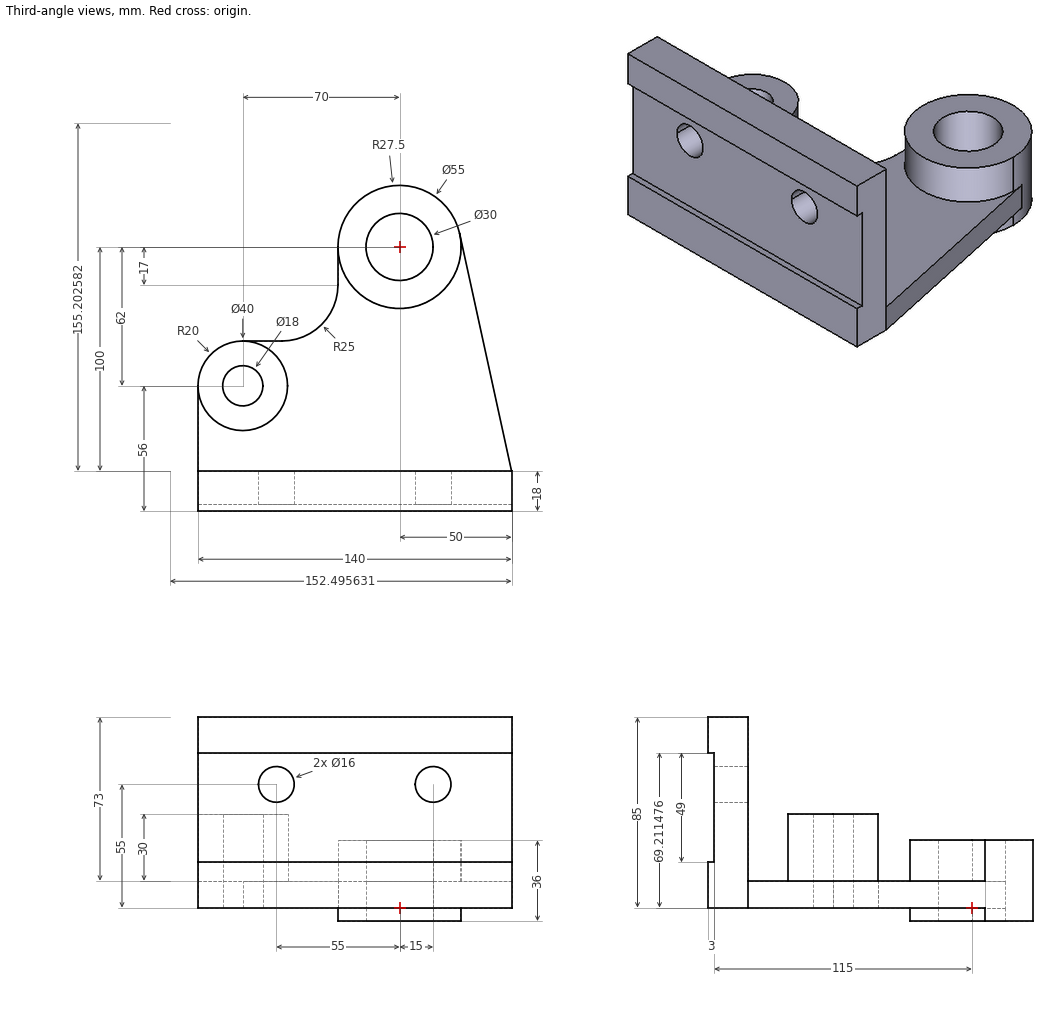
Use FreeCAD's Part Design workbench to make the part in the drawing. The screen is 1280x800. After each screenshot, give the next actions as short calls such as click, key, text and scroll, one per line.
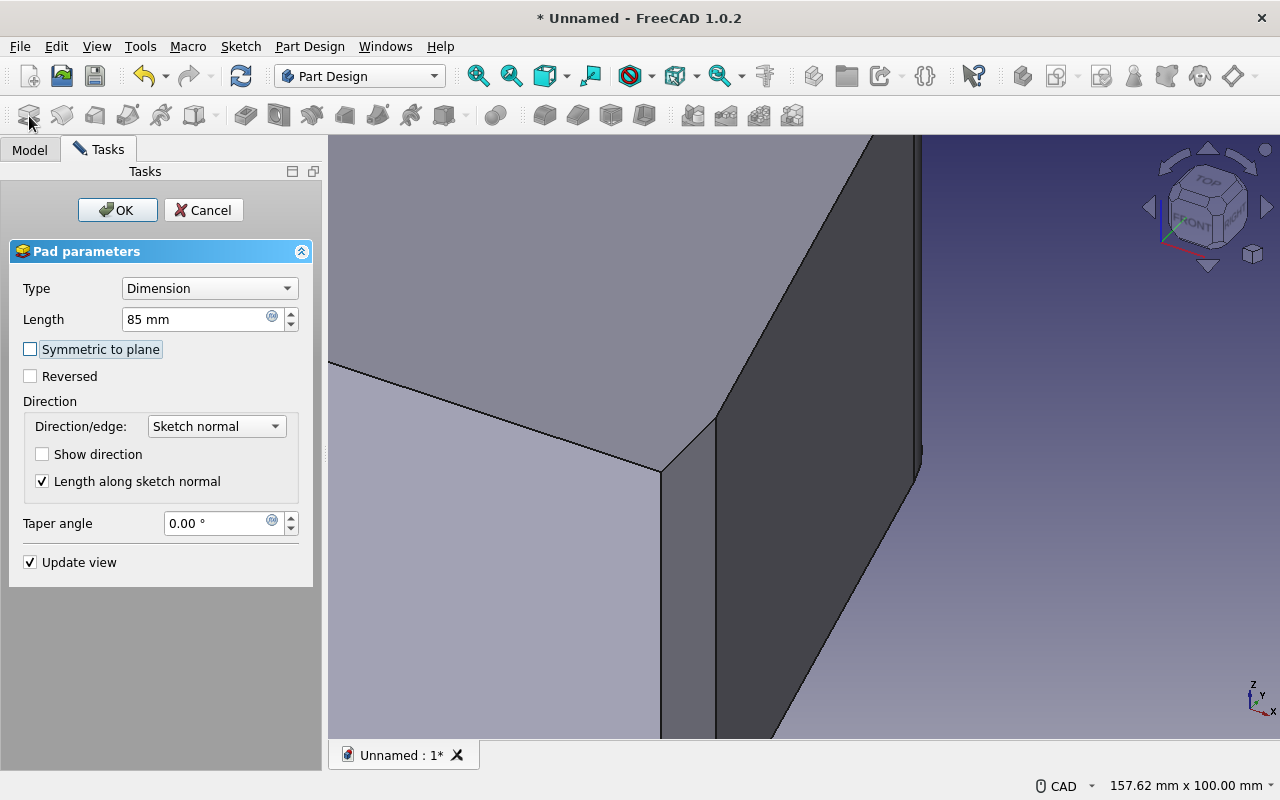
click(118, 210)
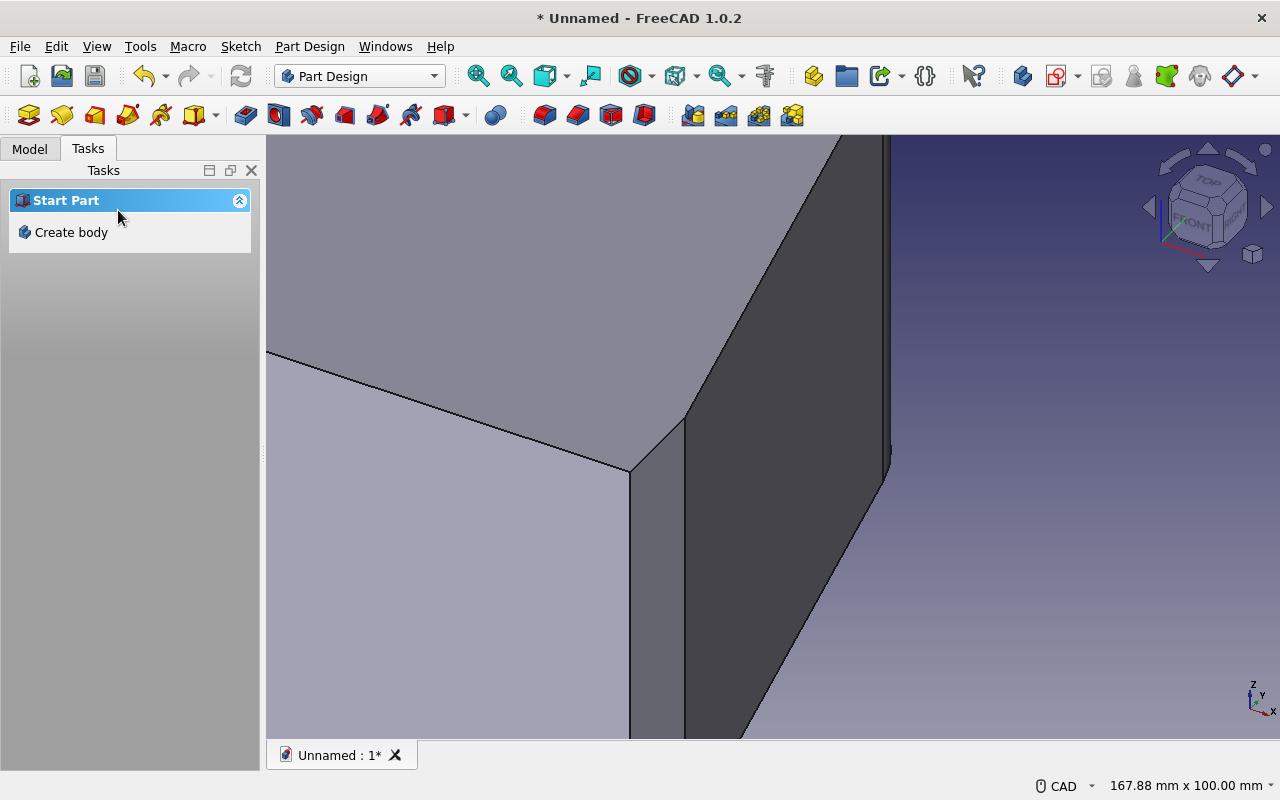
click(479, 76)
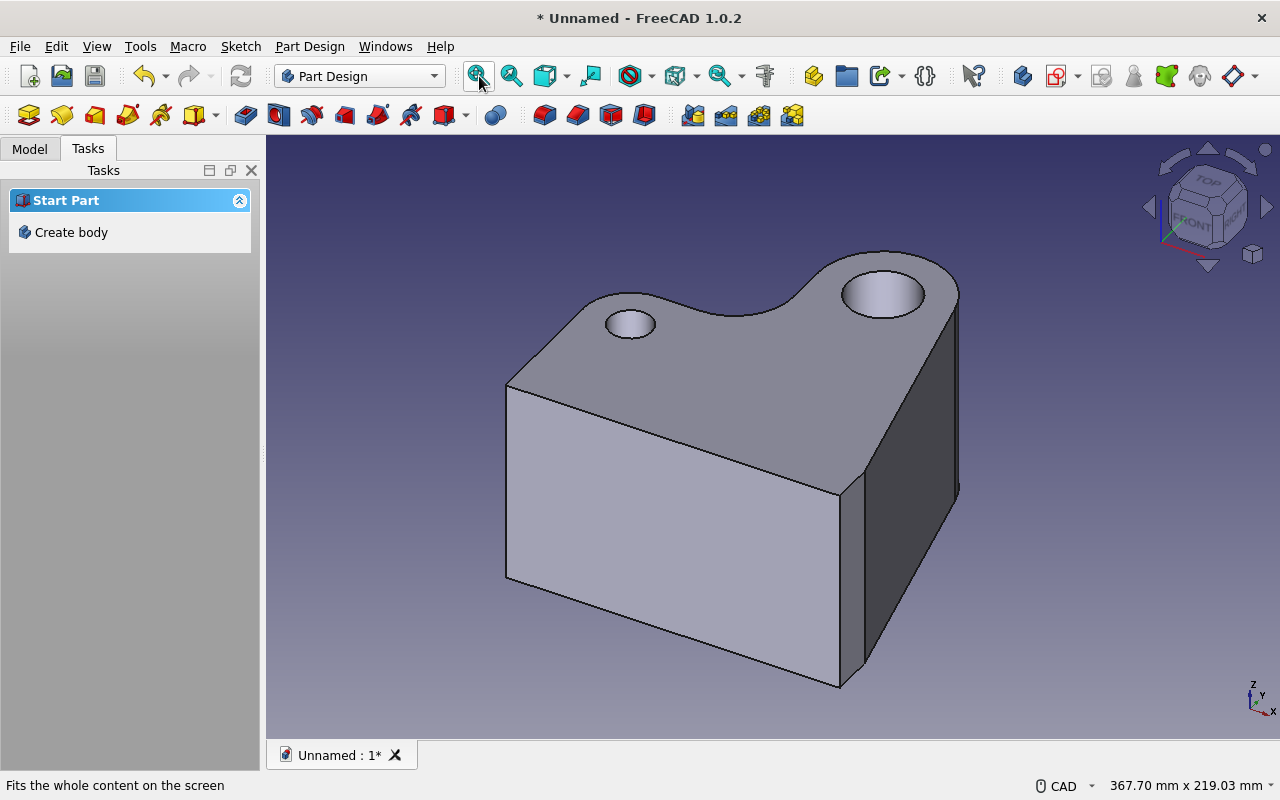
click(792, 384)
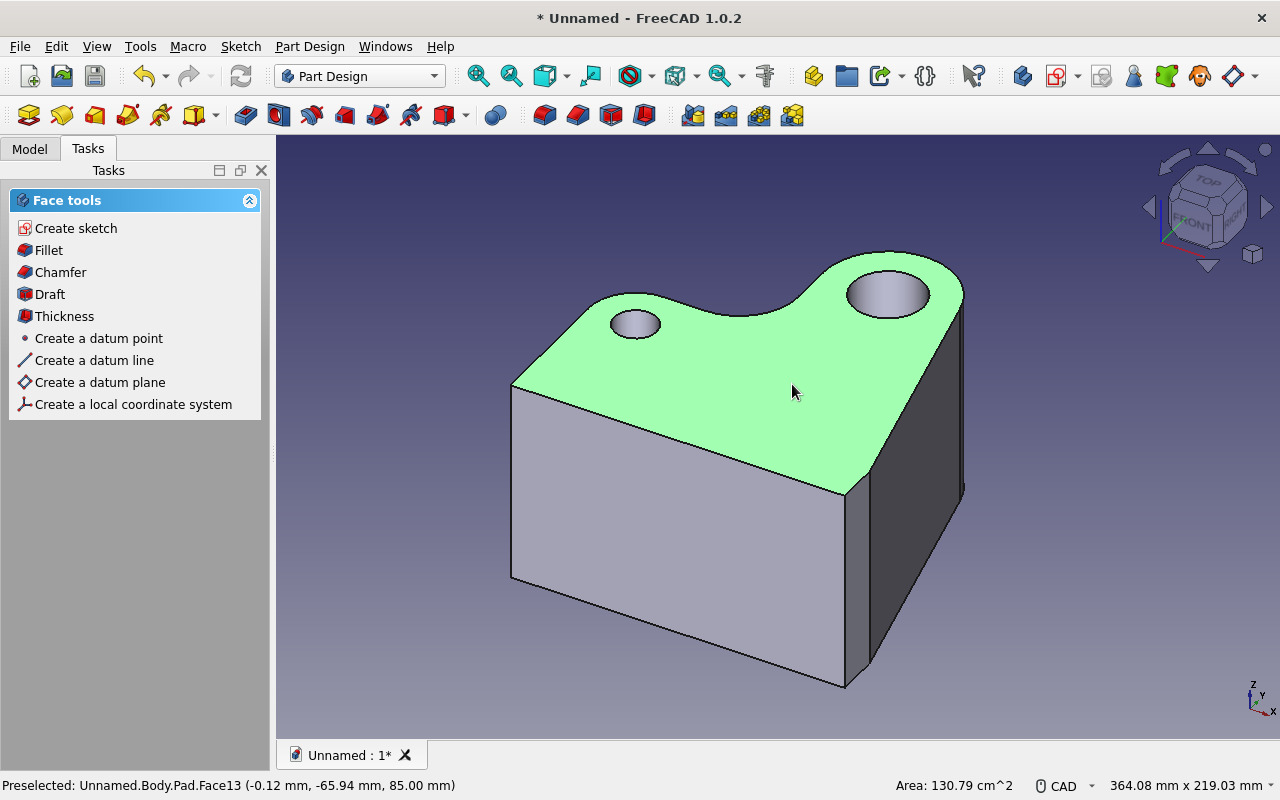
click(1056, 76)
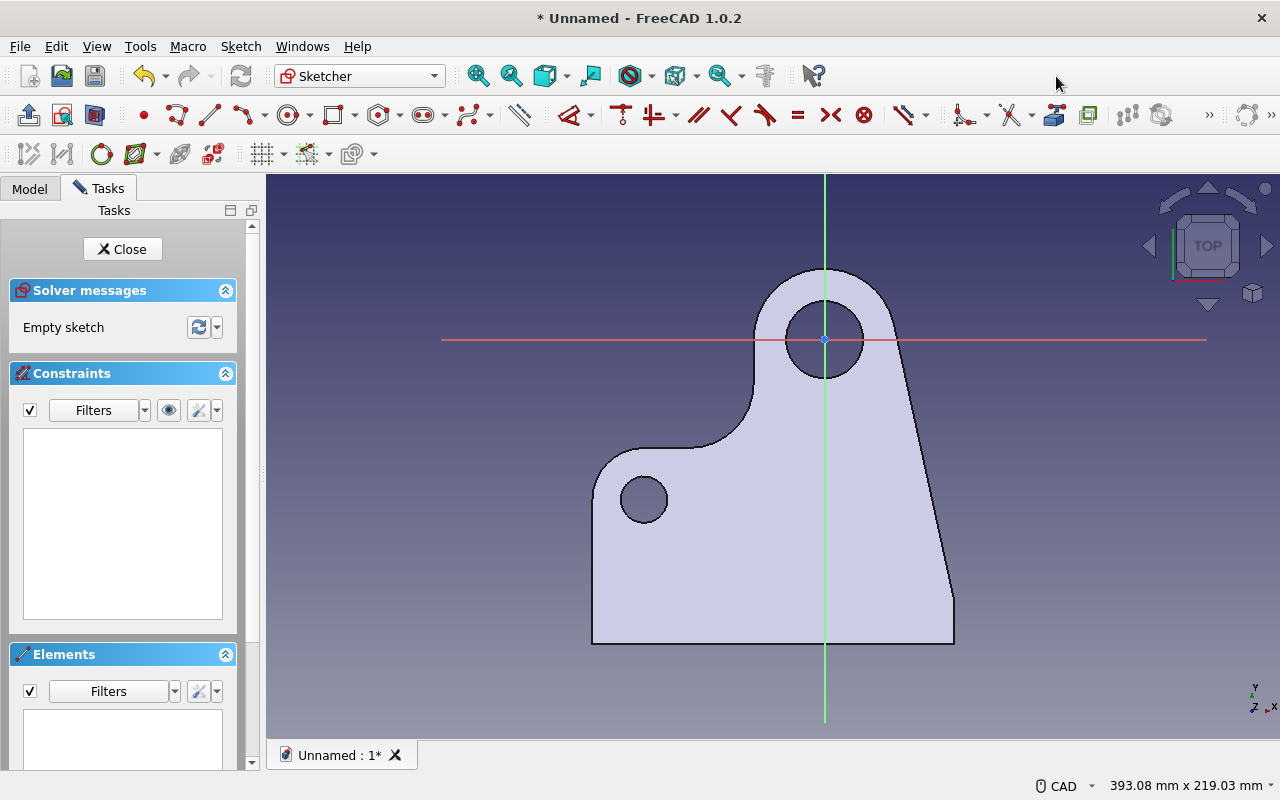
scroll(468, 711, down, 1)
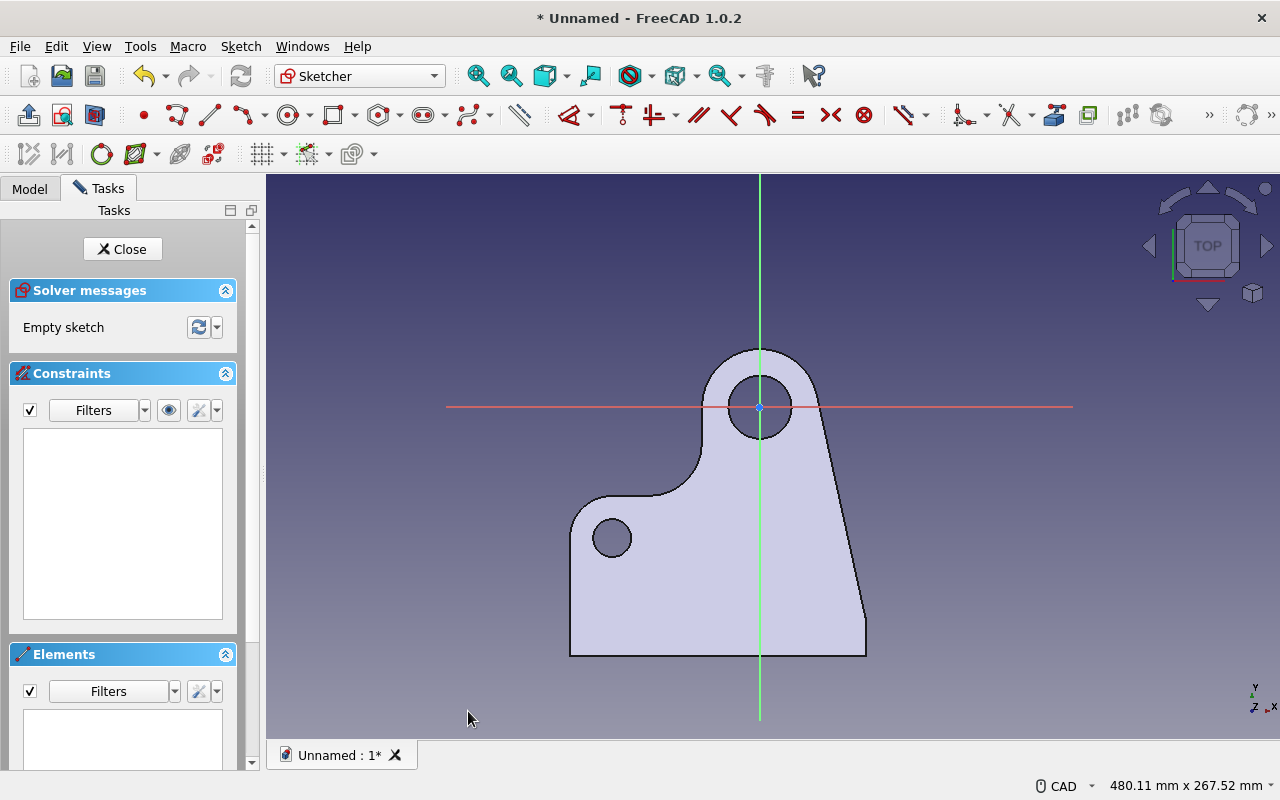
click(332, 116)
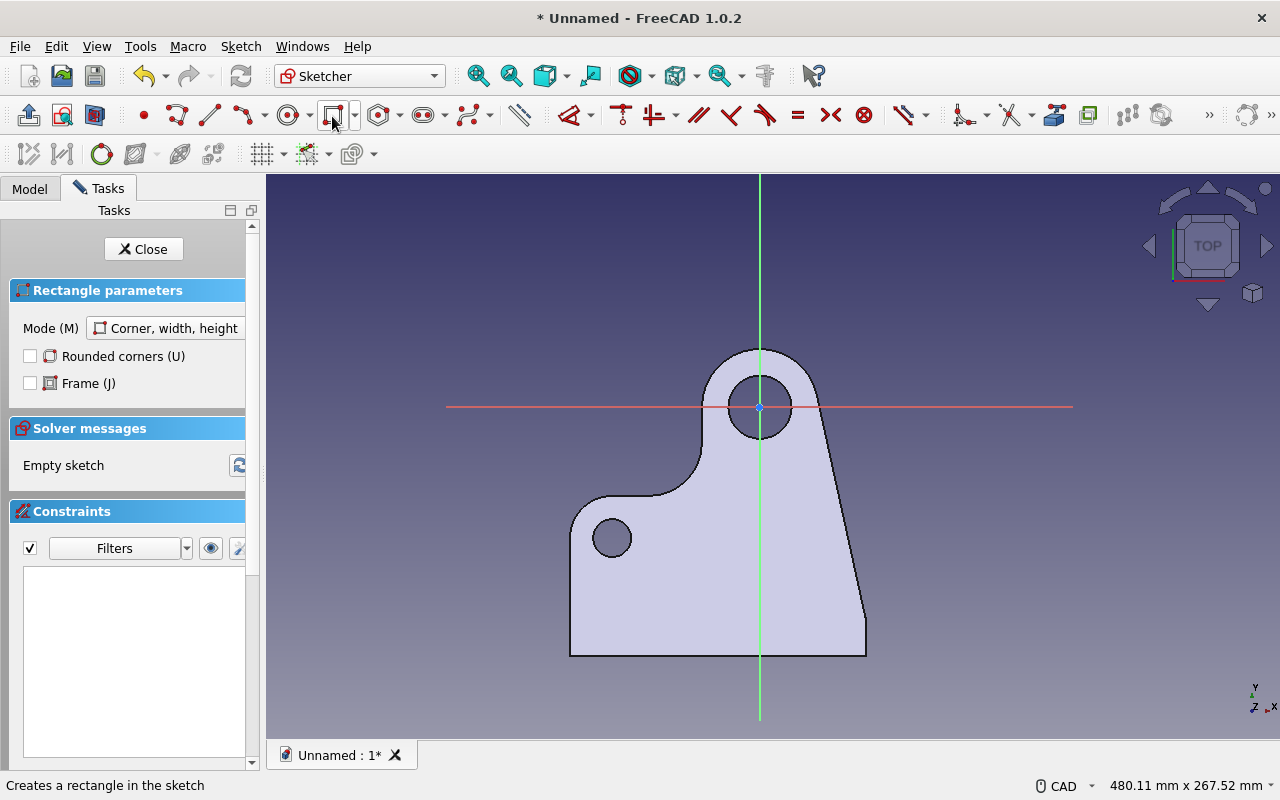
click(544, 291)
click(866, 618)
key(Escape)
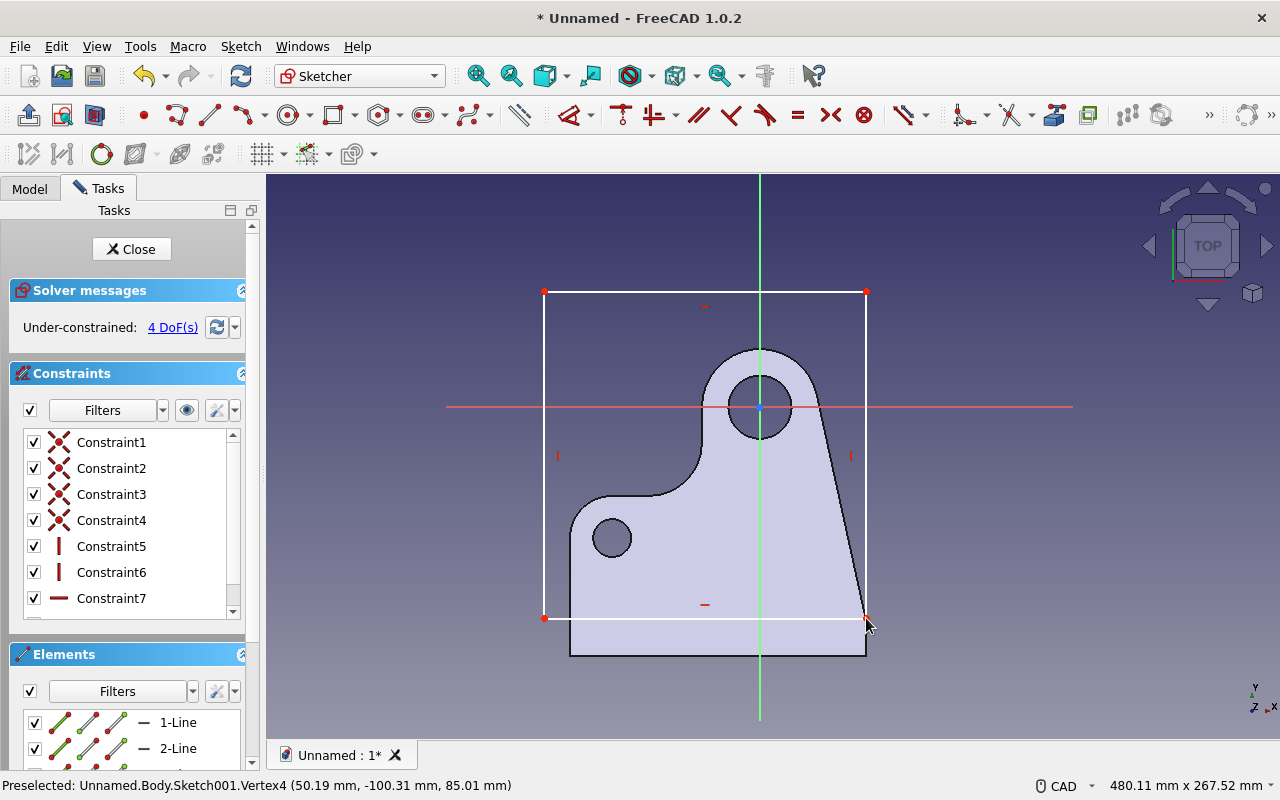
key(d)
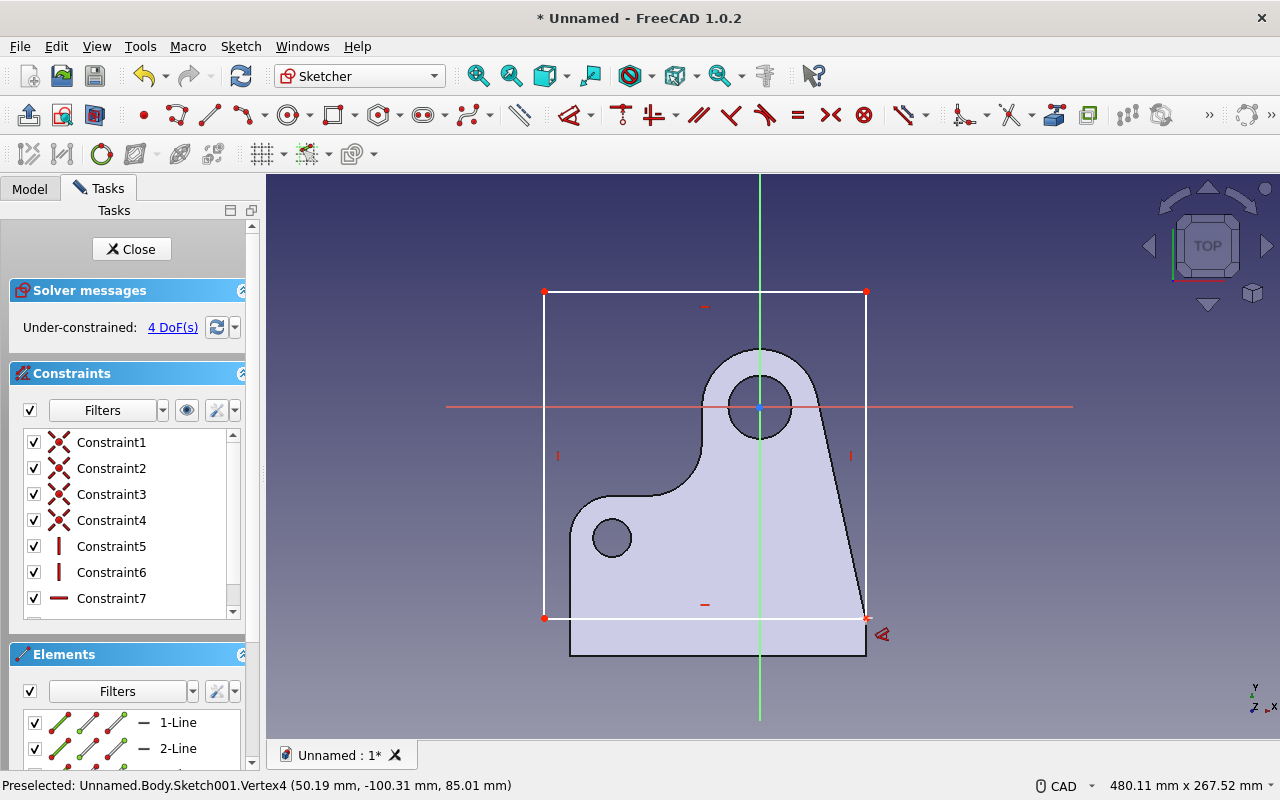
click(866, 619)
click(813, 653)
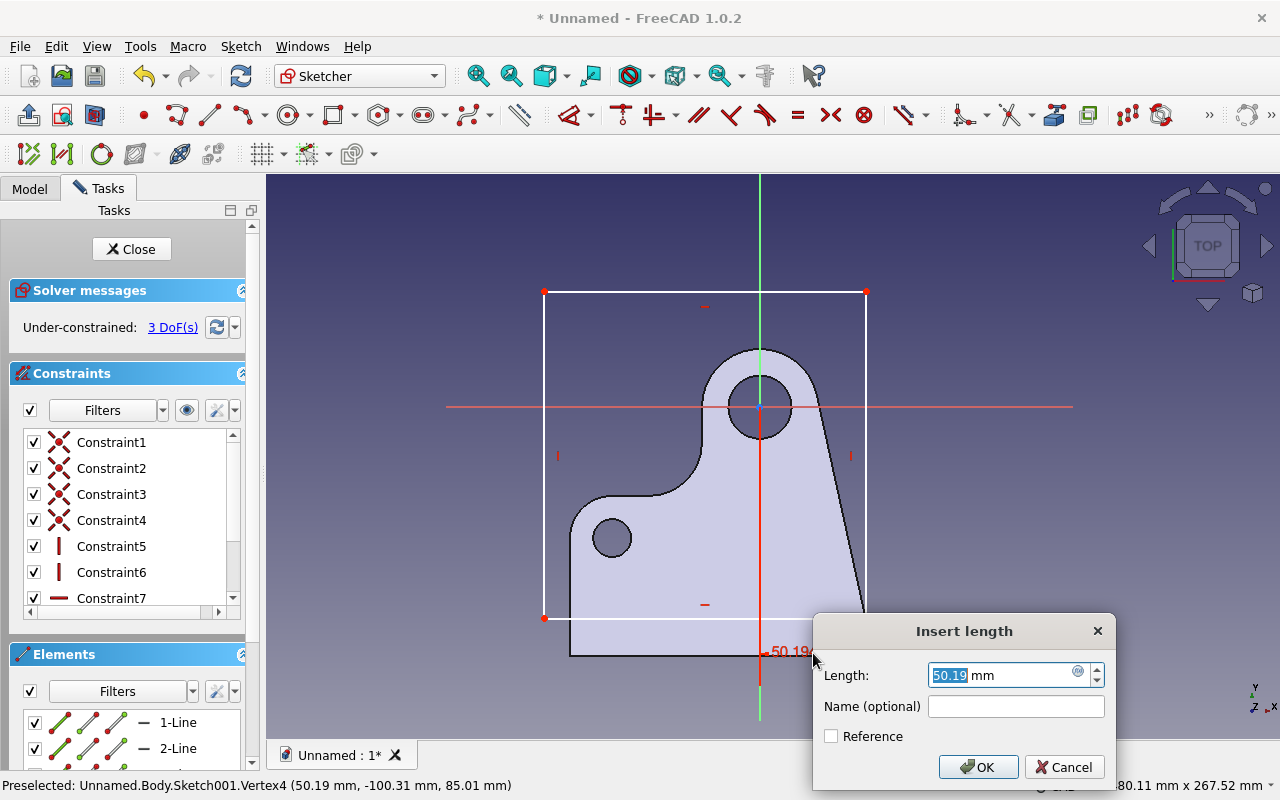
text(50)
key(Return)